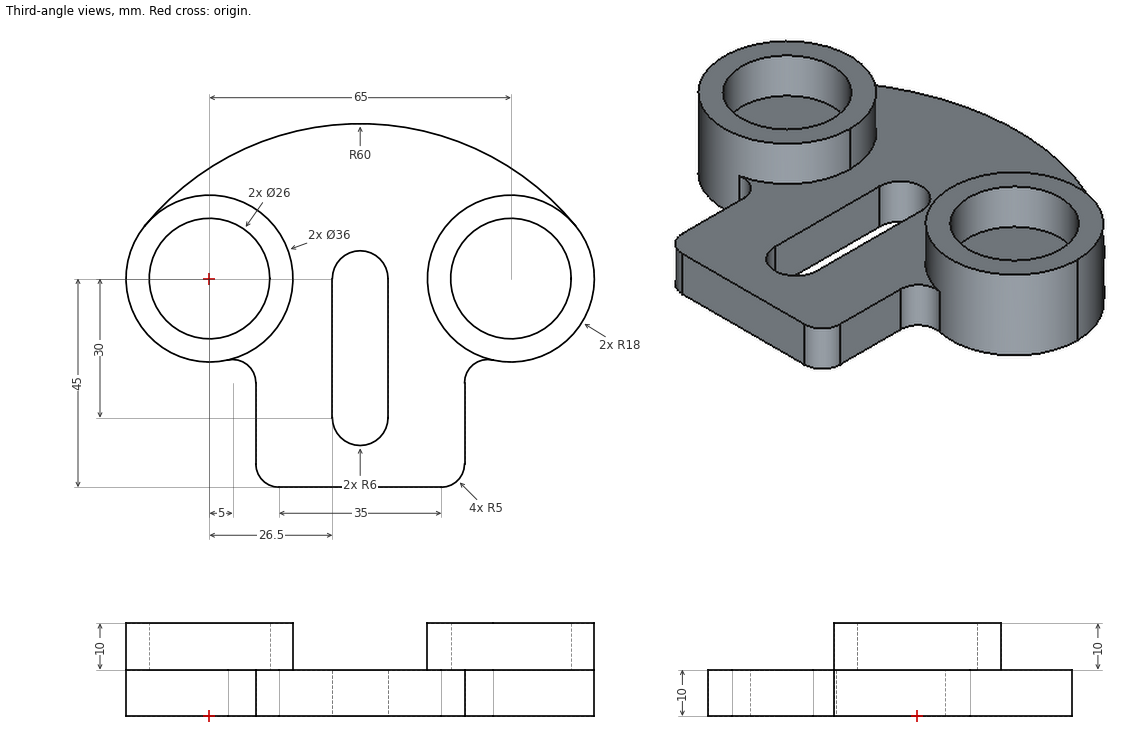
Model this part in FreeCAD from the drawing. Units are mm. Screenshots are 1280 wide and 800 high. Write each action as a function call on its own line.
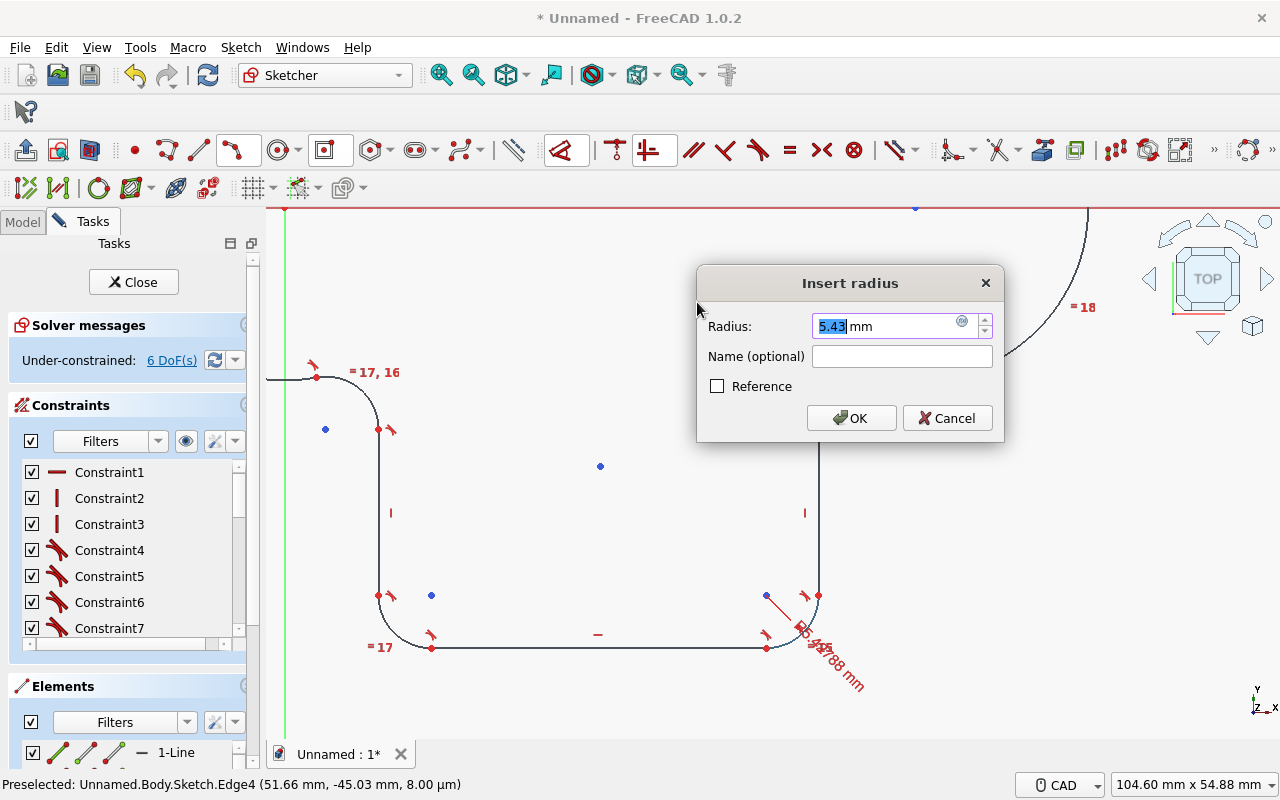
text(5)
key(Return)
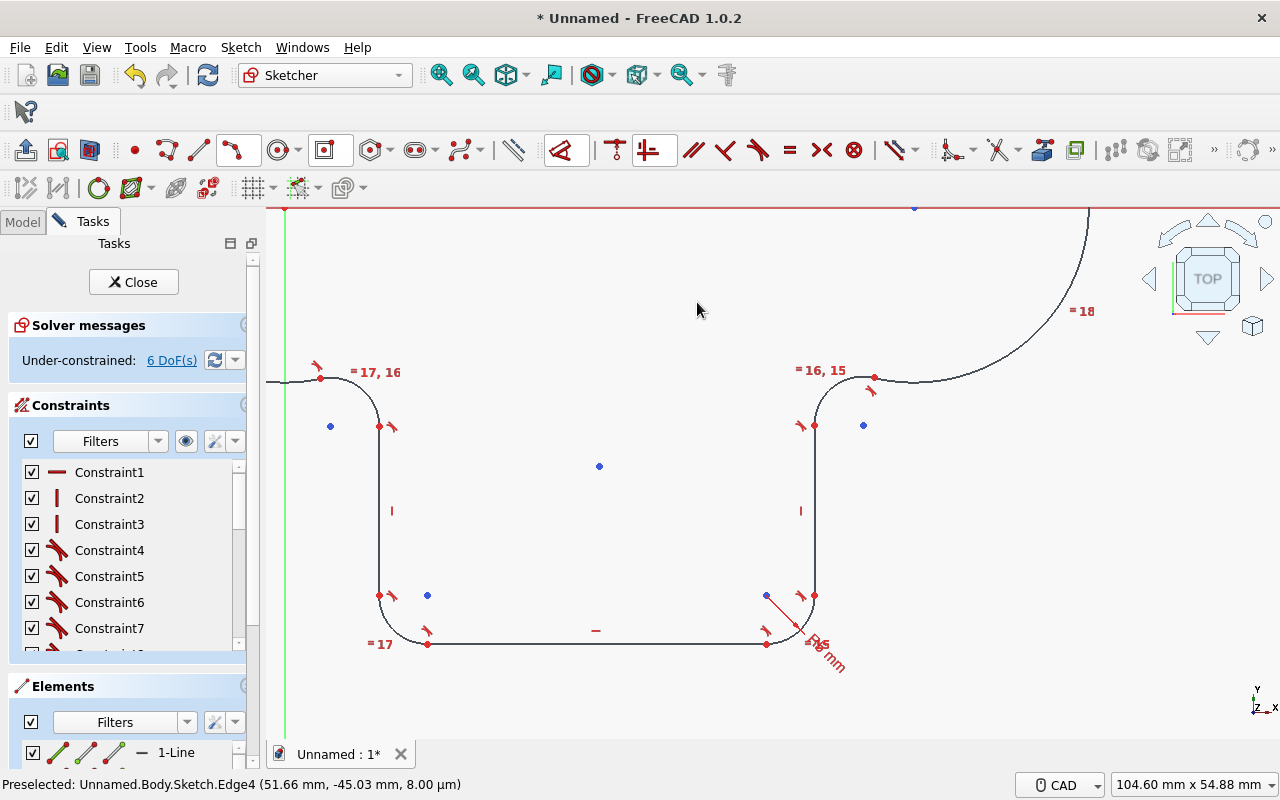
click(1000, 360)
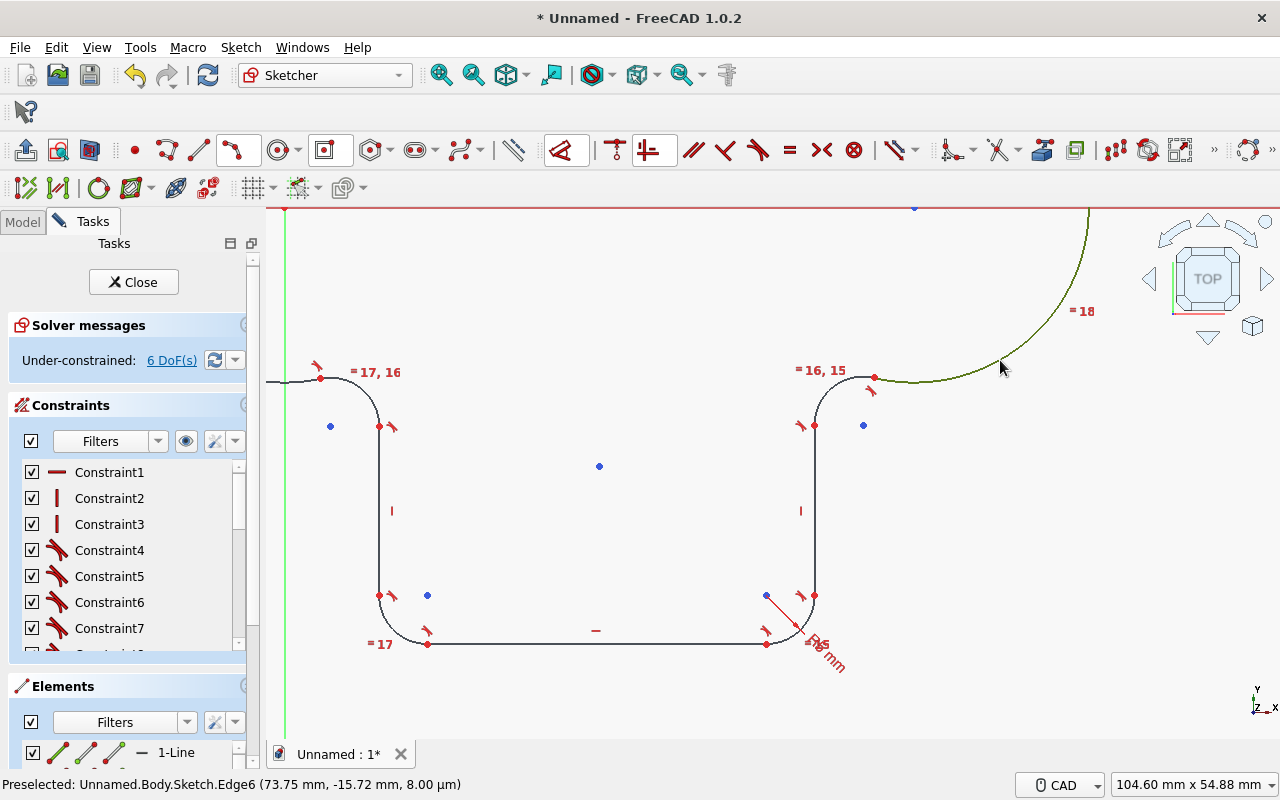
key(k)
key(r)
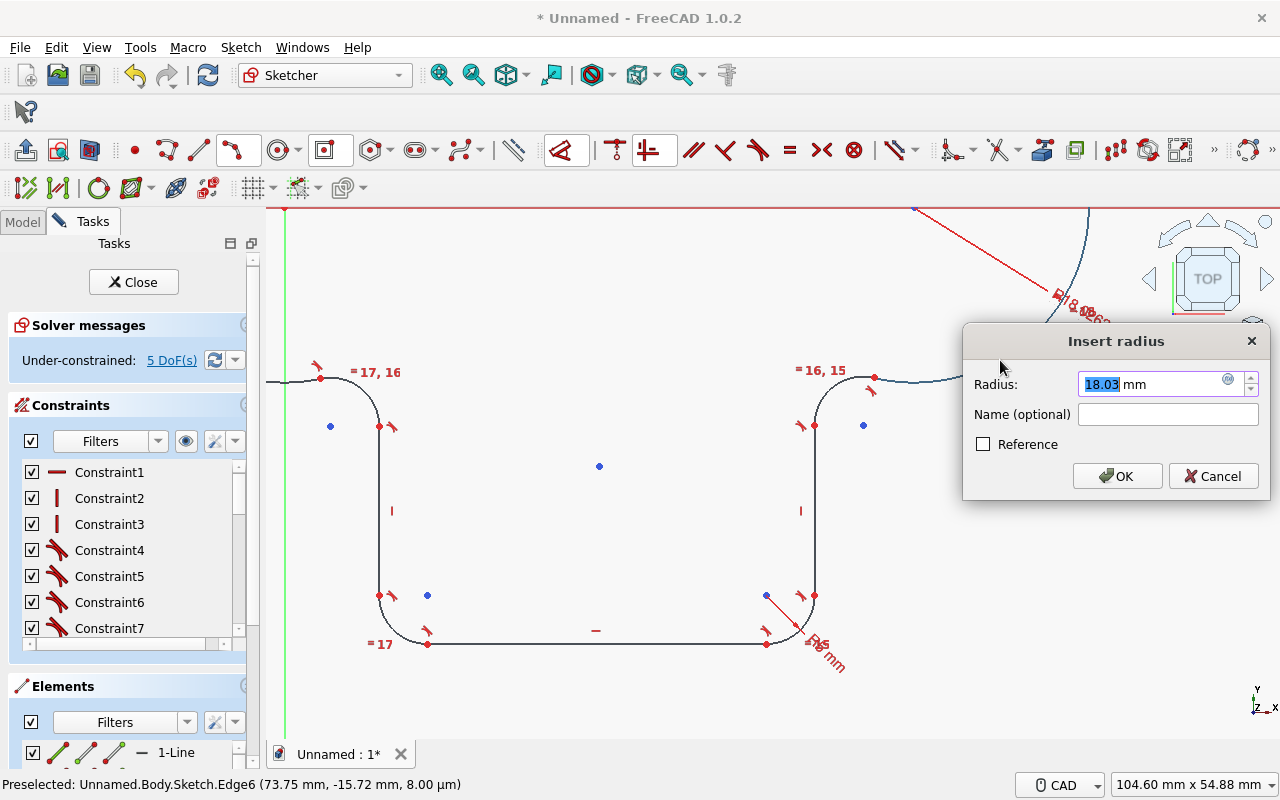
text(18)
key(Return)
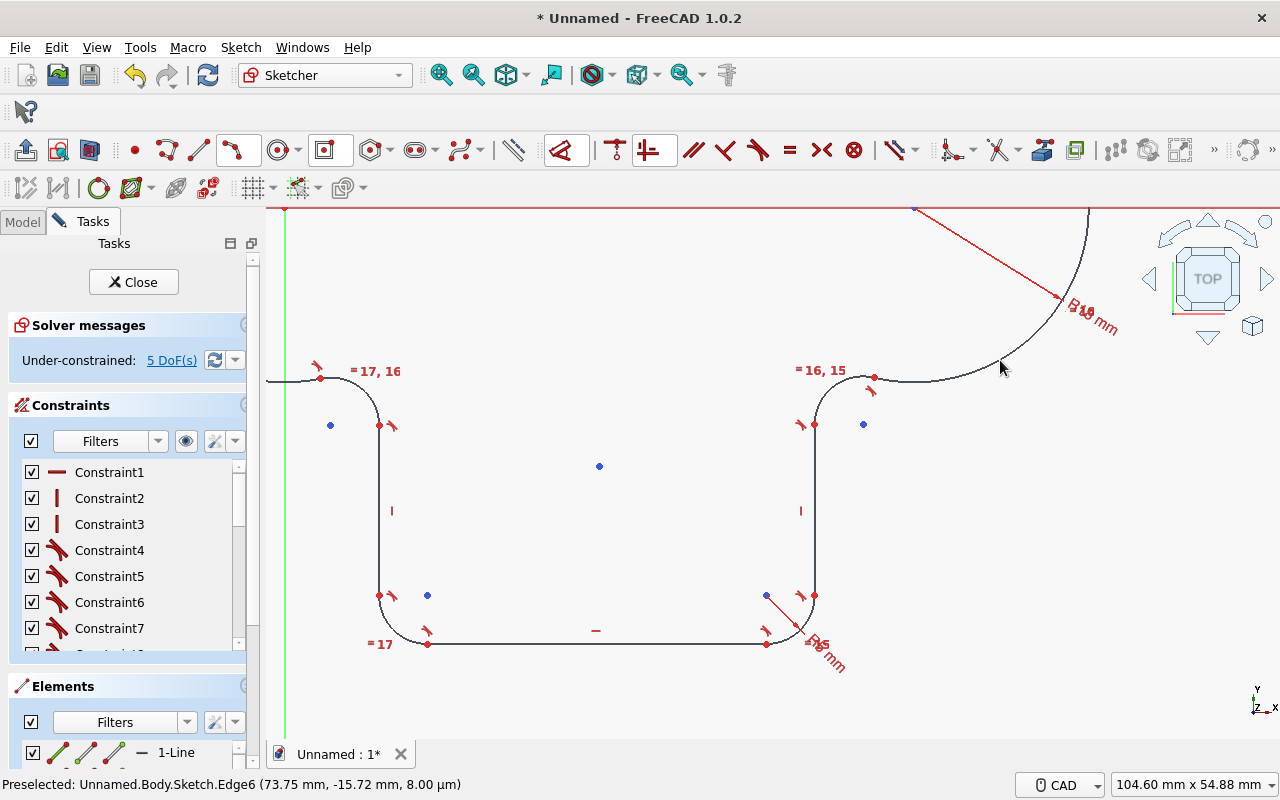
scroll(790, 643, down, 4)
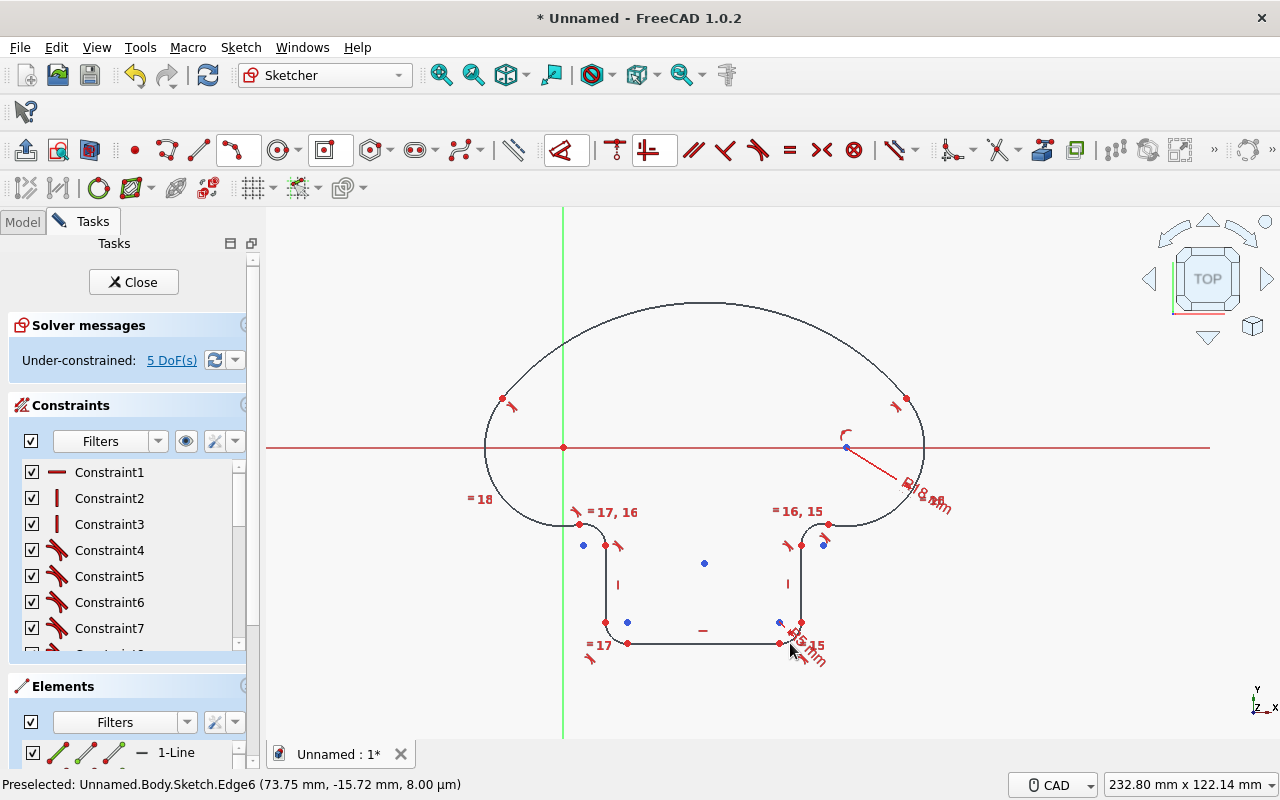
click(795, 319)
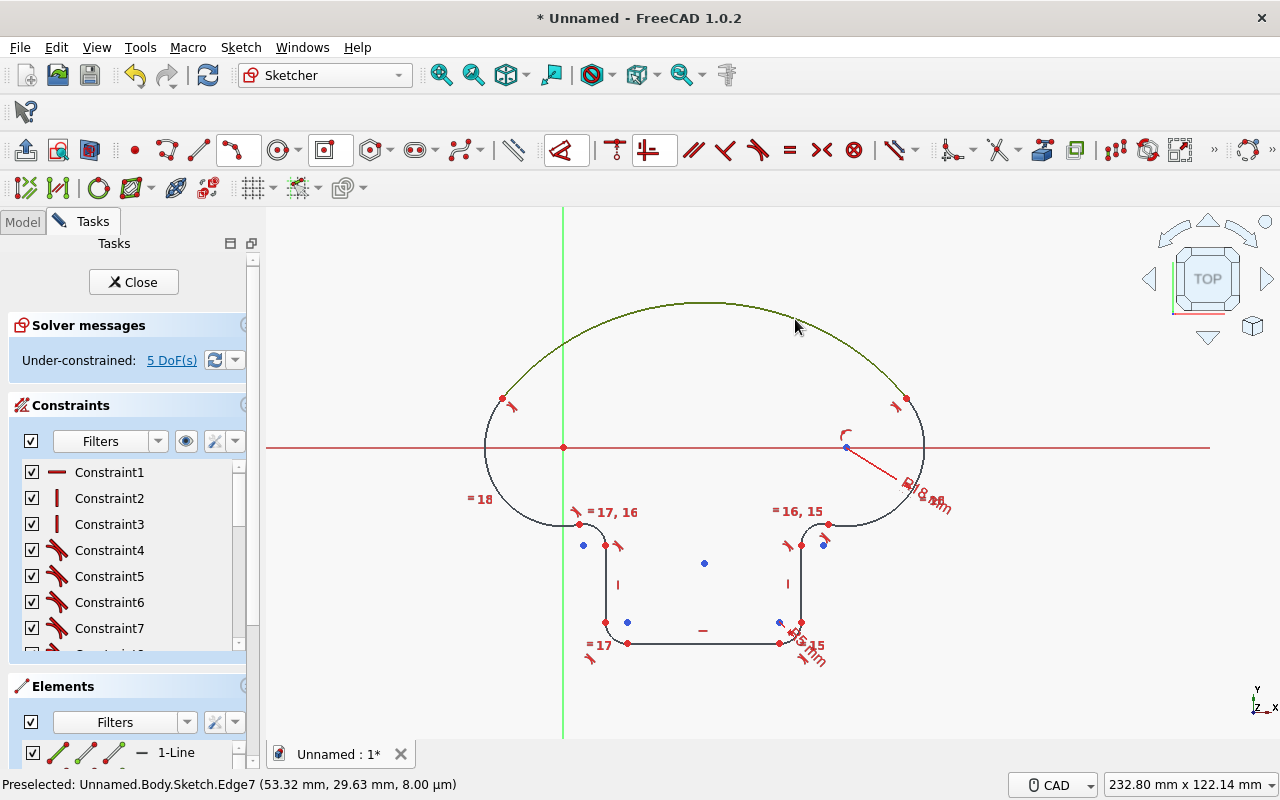
click(584, 150)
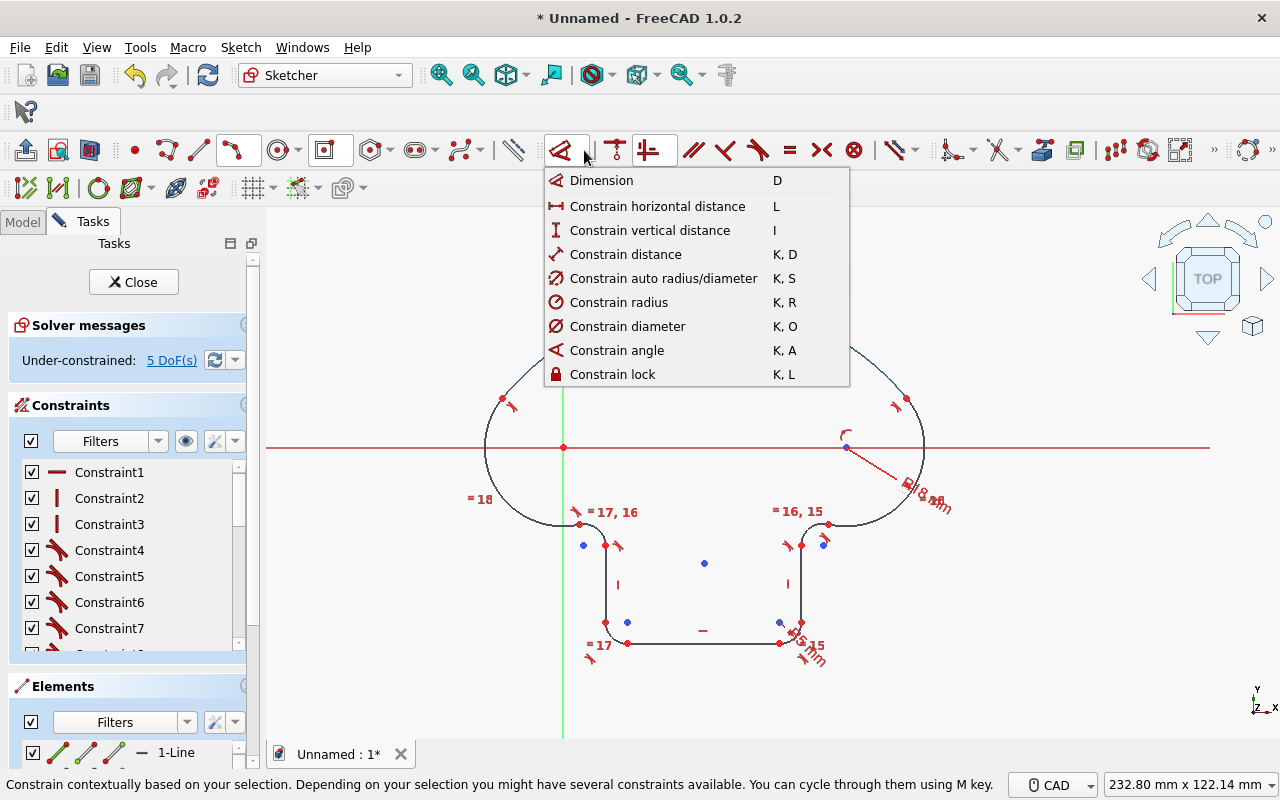
click(697, 302)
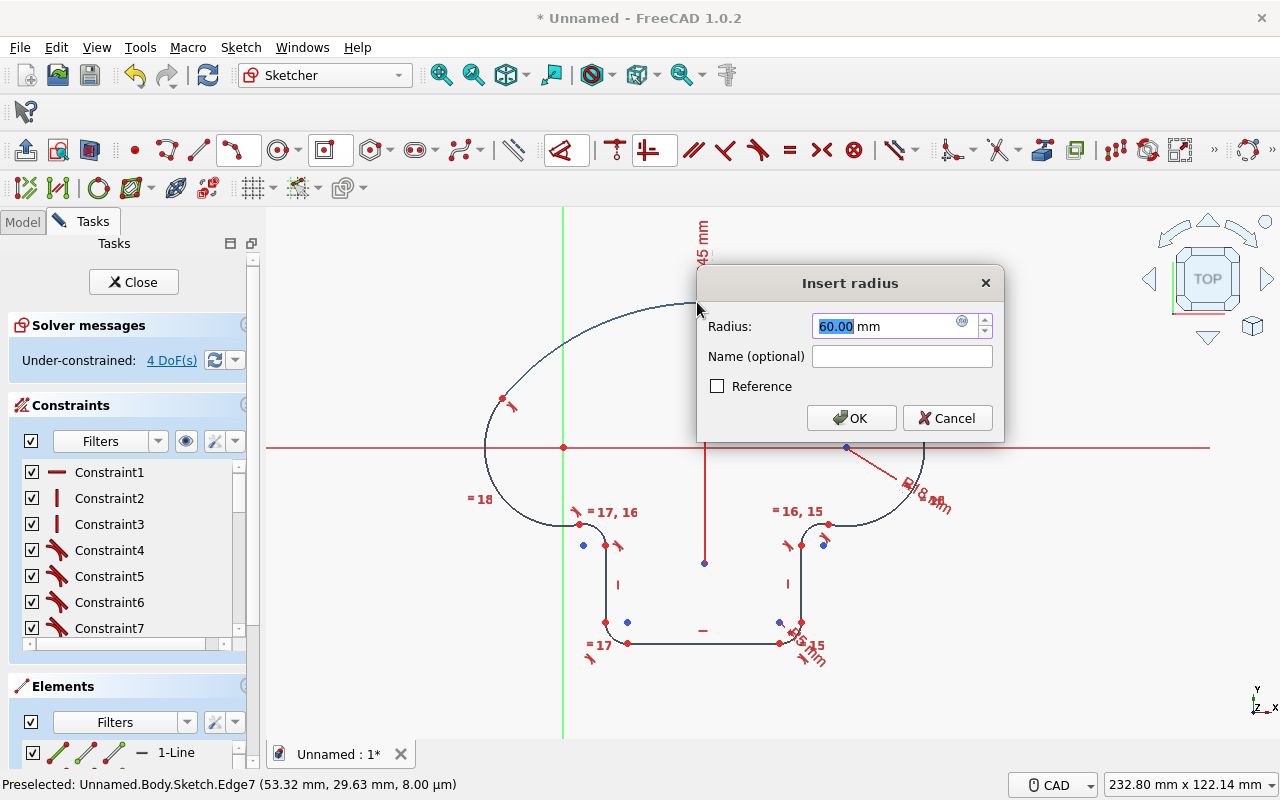
text(60)
key(Return)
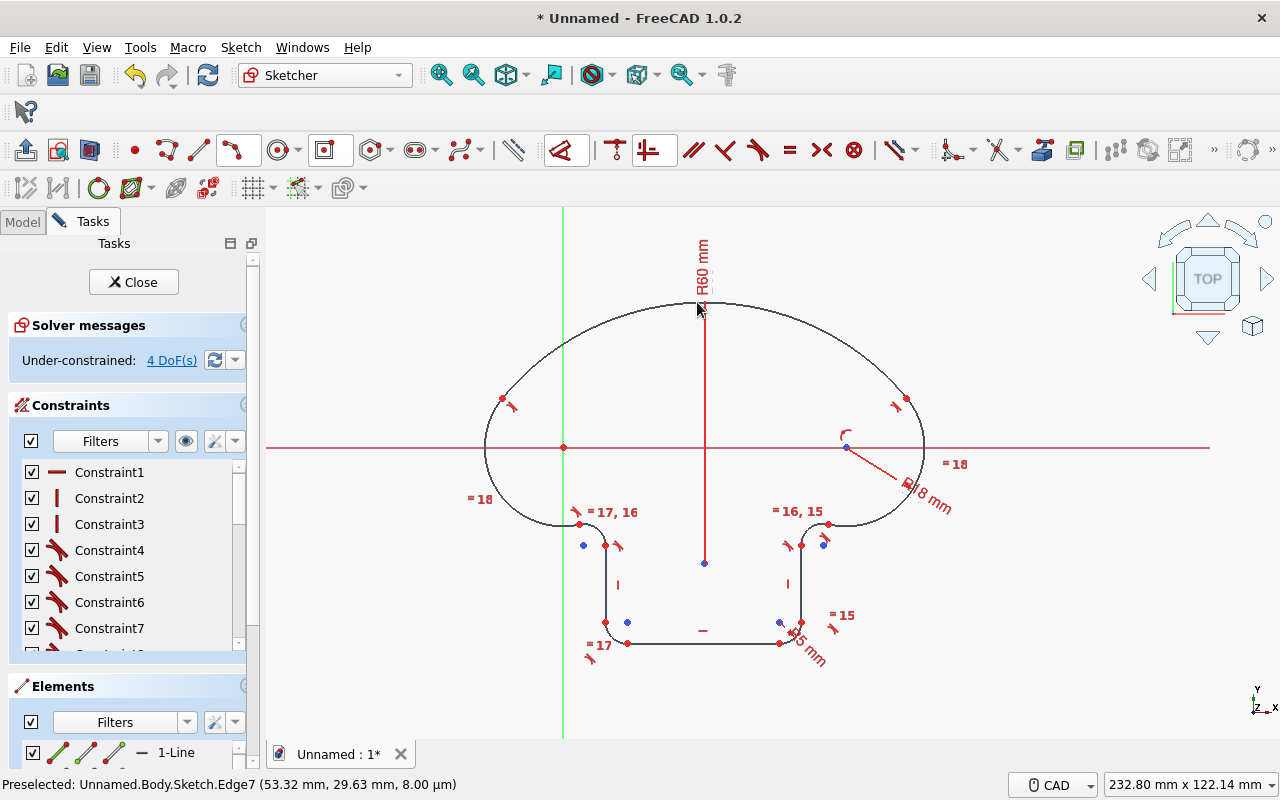
click(673, 644)